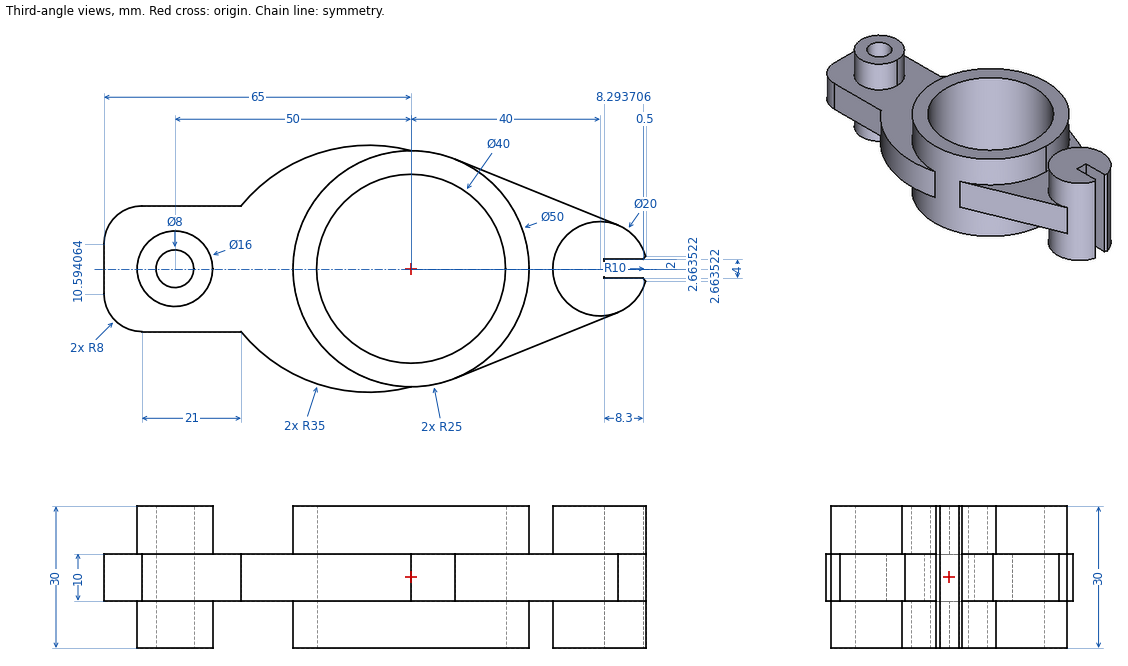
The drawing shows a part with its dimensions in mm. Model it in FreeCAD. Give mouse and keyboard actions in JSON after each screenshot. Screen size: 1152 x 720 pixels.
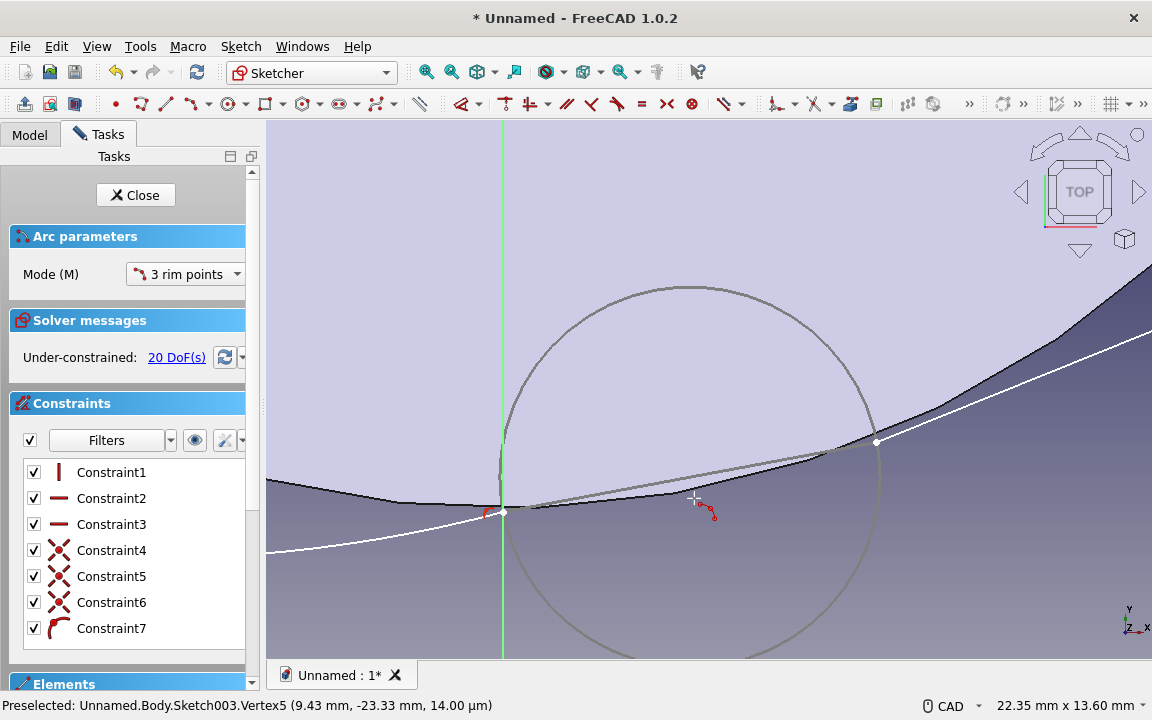
{"action": "left_click", "coordinate": [692, 490]}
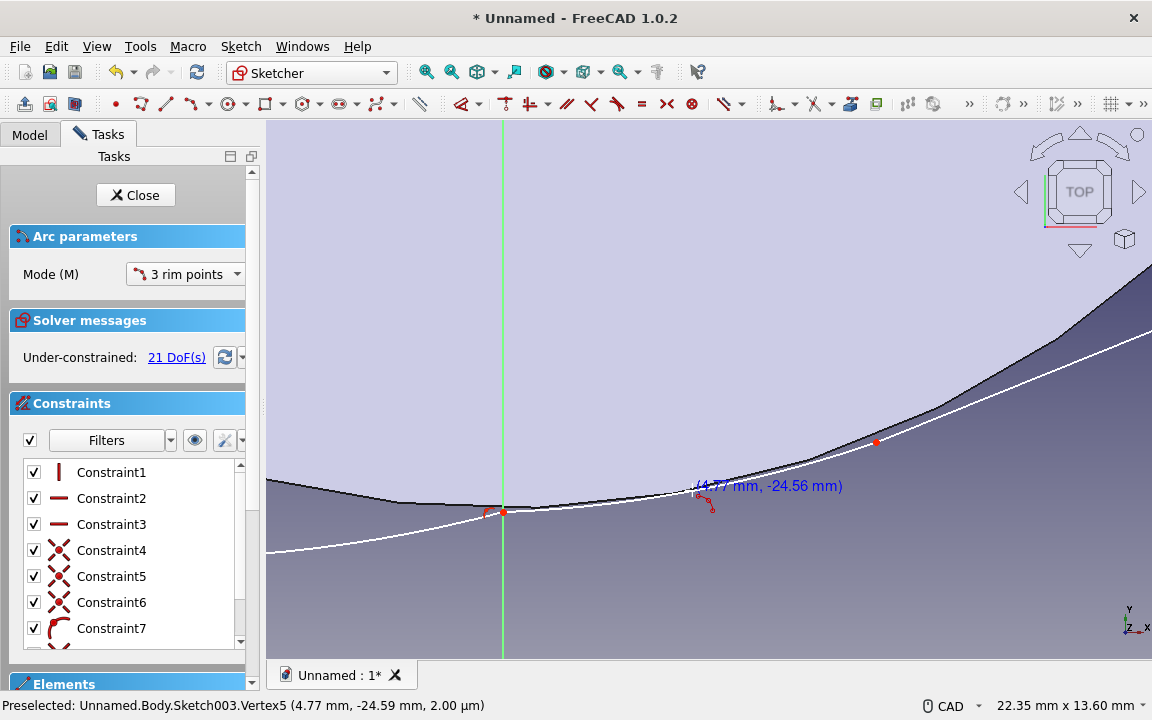
{"action": "scroll", "coordinate": [695, 498], "scroll_direction": "down", "scroll_amount": 11}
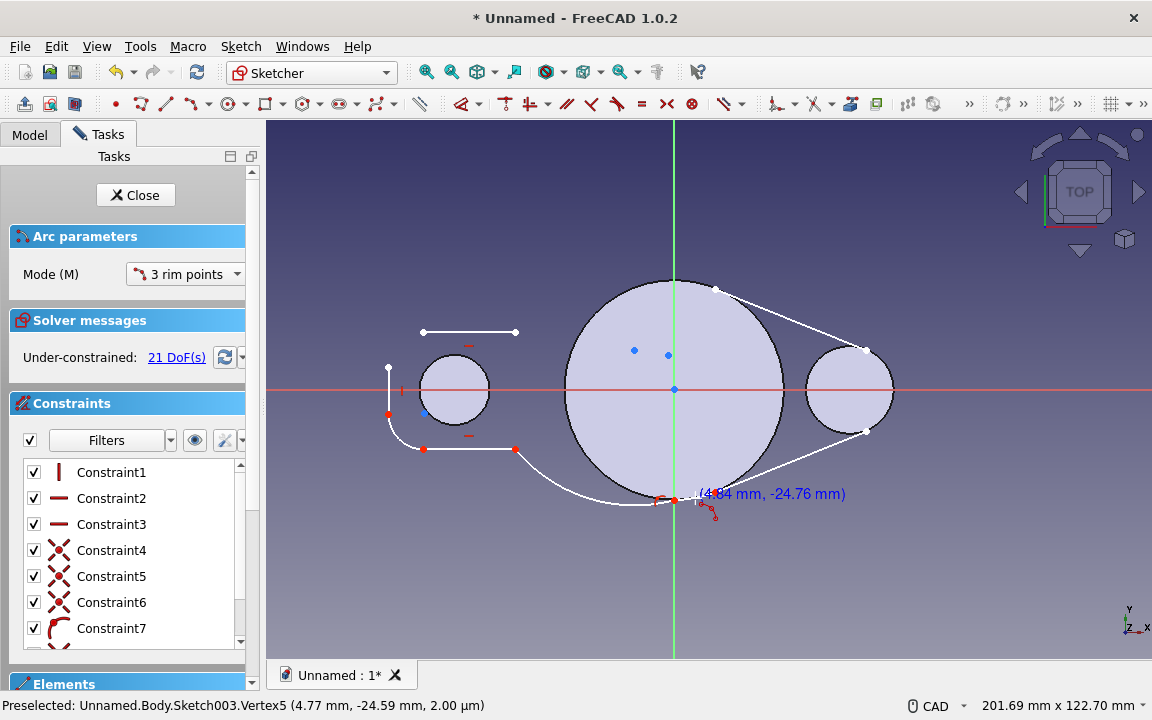
{"action": "left_click", "coordinate": [867, 431]}
{"action": "left_click", "coordinate": [867, 350]}
{"action": "left_click", "coordinate": [889, 410]}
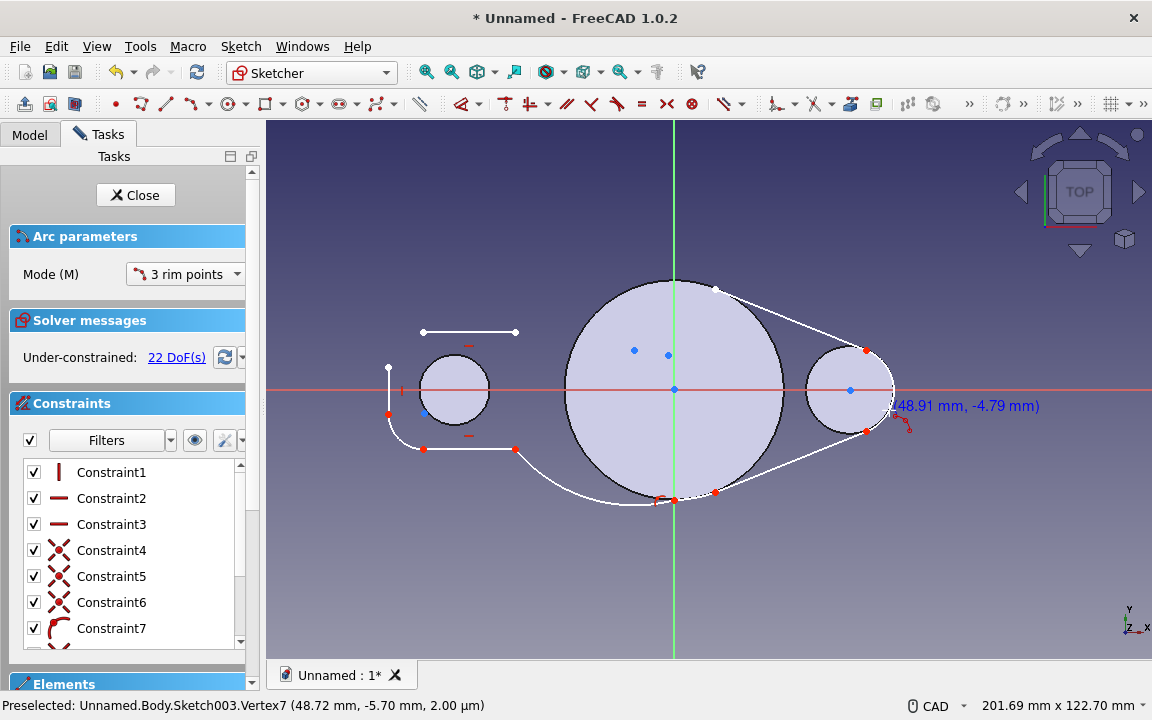
{"action": "left_click", "coordinate": [716, 289]}
{"action": "left_click", "coordinate": [674, 280]}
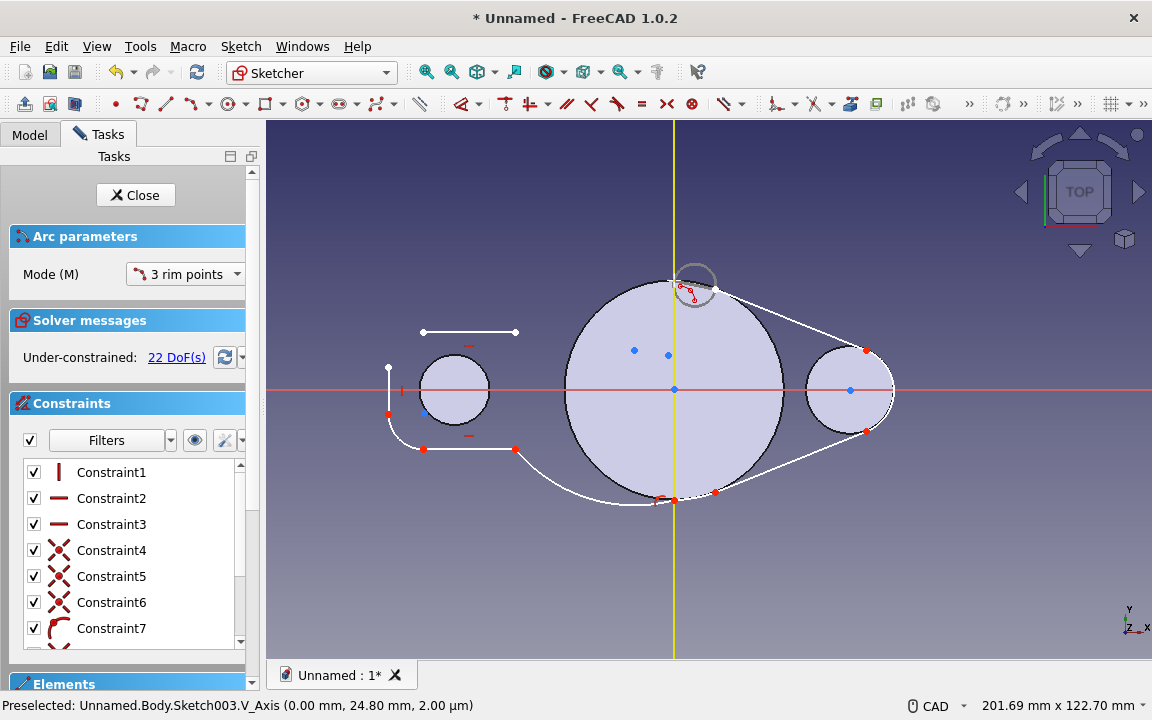
{"action": "scroll", "coordinate": [695, 282], "scroll_direction": "up", "scroll_amount": 11}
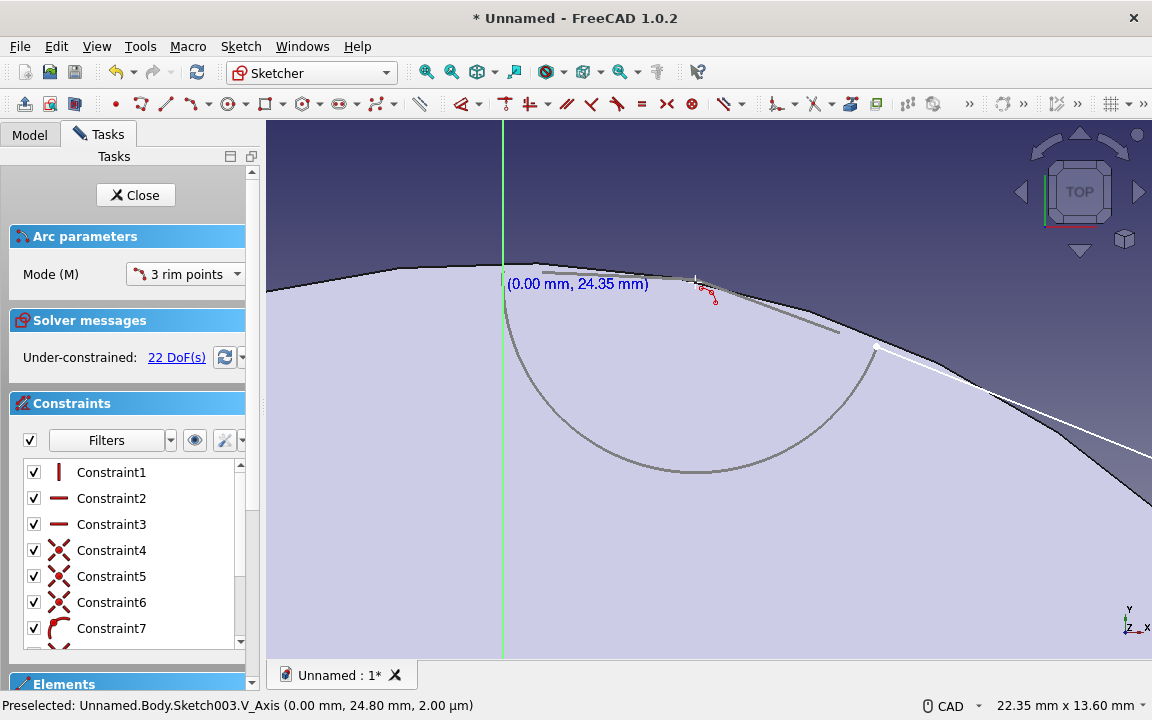
{"action": "left_click", "coordinate": [692, 281]}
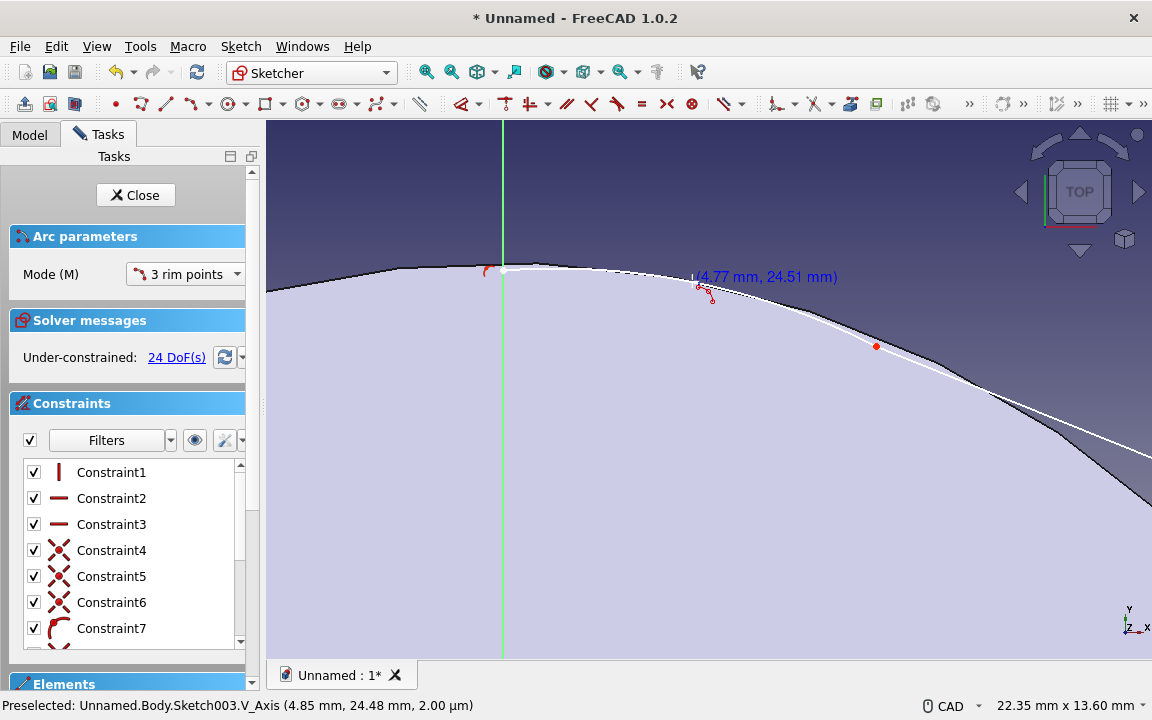
{"action": "scroll", "coordinate": [695, 282], "scroll_direction": "down", "scroll_amount": 11}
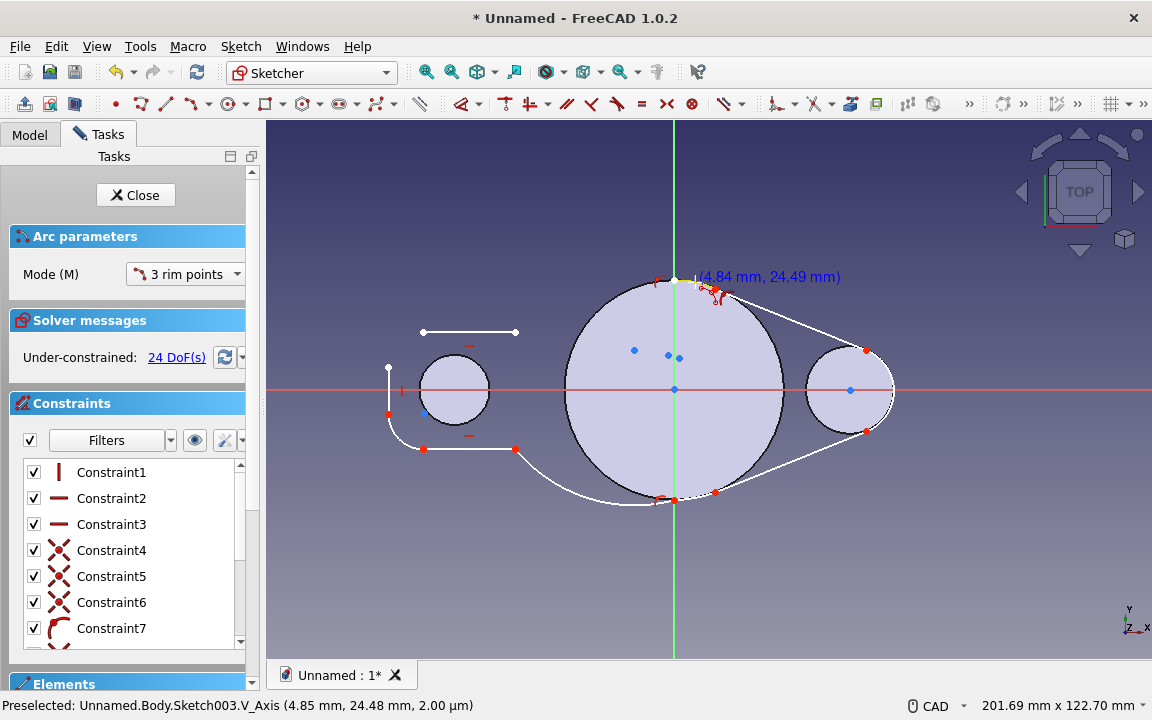
{"action": "left_click", "coordinate": [674, 281]}
{"action": "left_click", "coordinate": [516, 332]}
{"action": "left_click", "coordinate": [588, 283]}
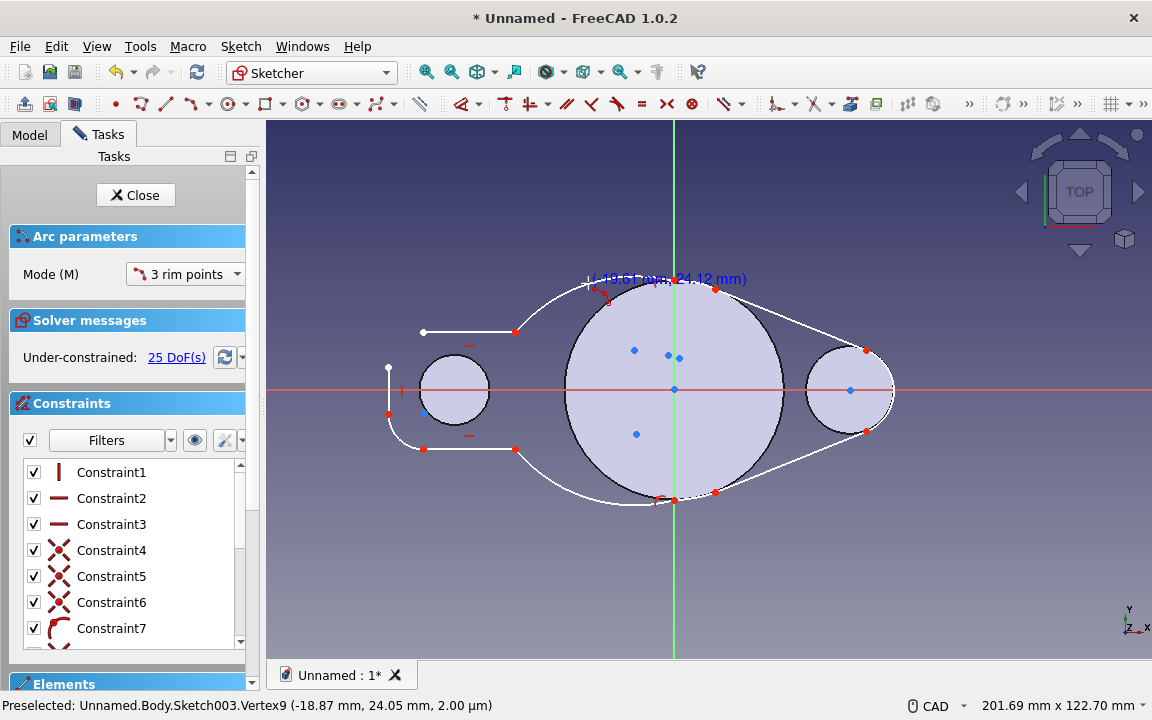
{"action": "left_click", "coordinate": [424, 332]}
{"action": "left_click", "coordinate": [389, 367]}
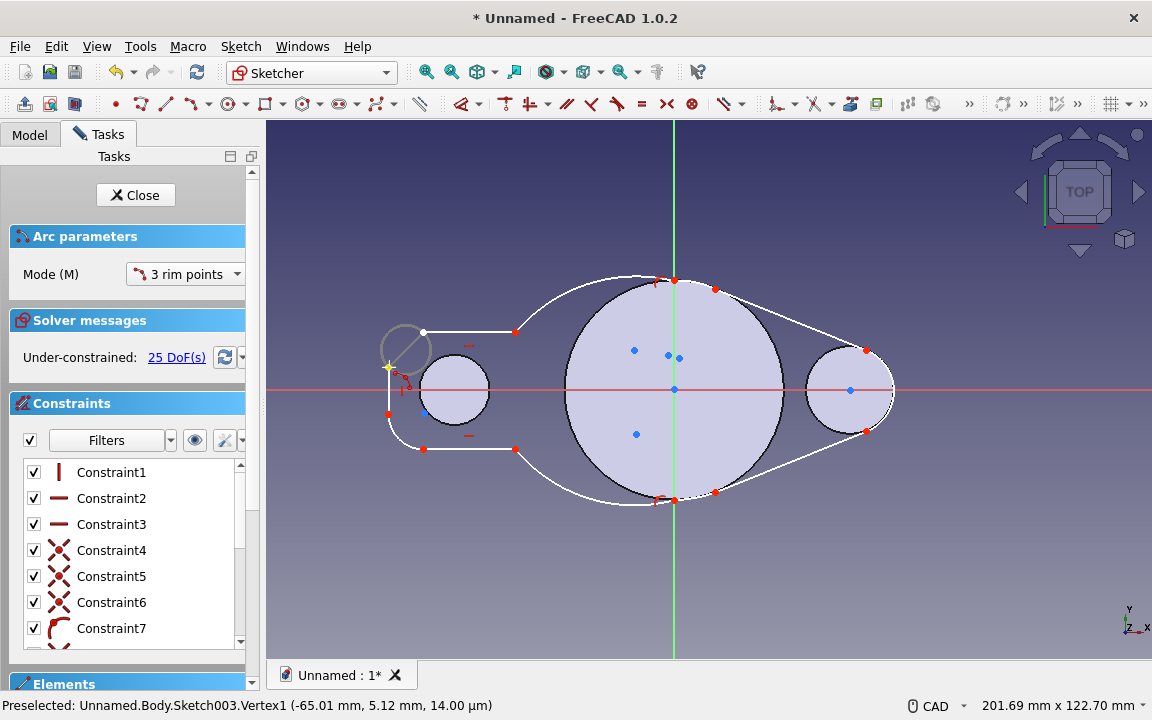
{"action": "scroll", "coordinate": [399, 342], "scroll_direction": "up", "scroll_amount": 3}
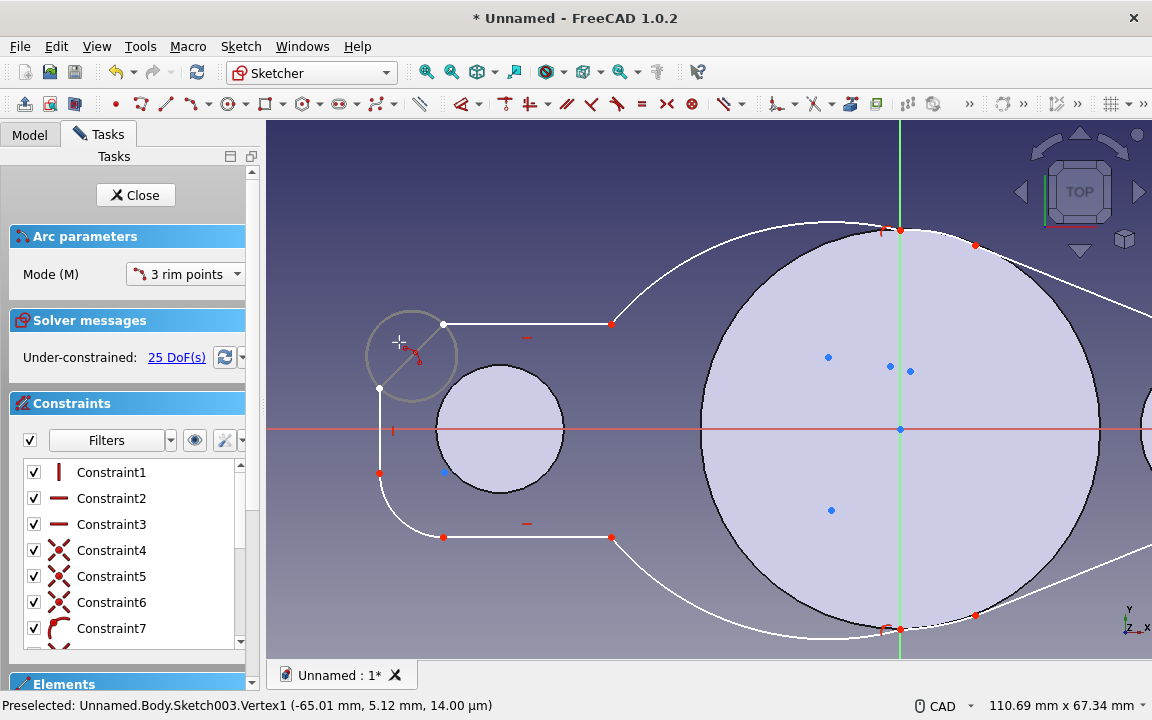
{"action": "left_click", "coordinate": [399, 341]}
{"action": "key", "text": "Escape"}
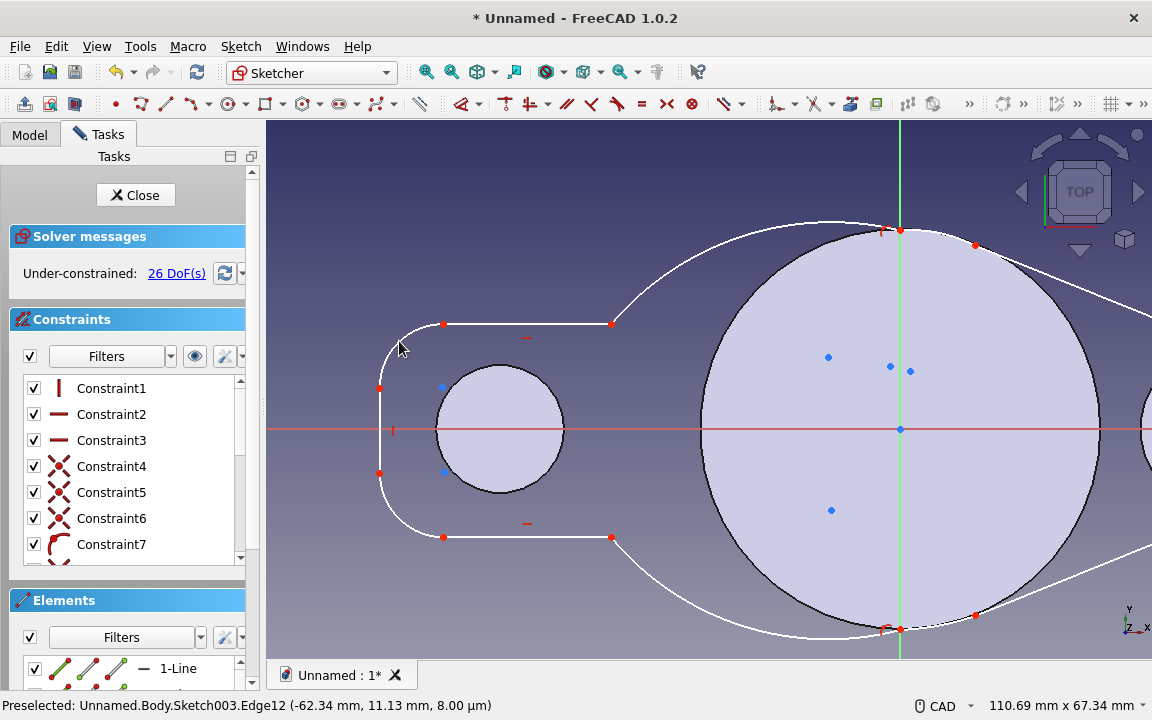
{"action": "left_click", "coordinate": [380, 414]}